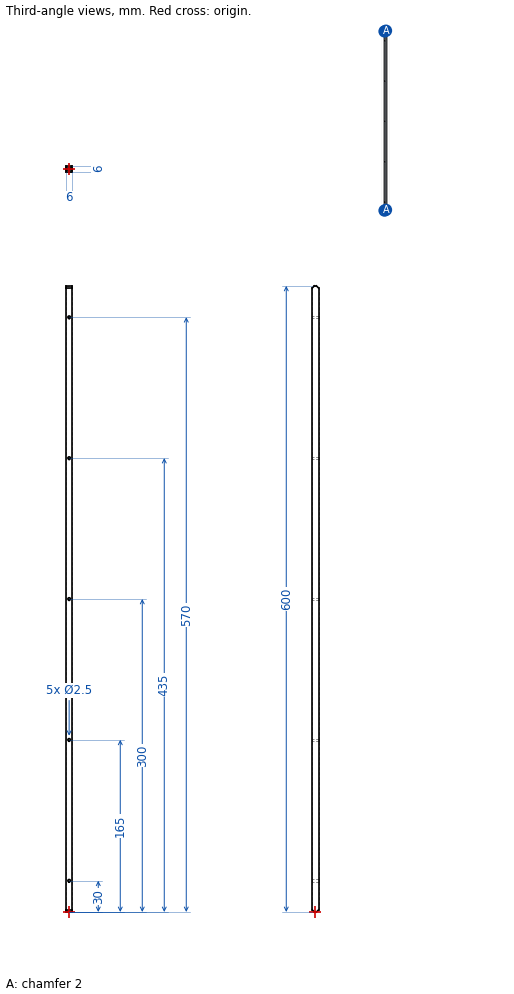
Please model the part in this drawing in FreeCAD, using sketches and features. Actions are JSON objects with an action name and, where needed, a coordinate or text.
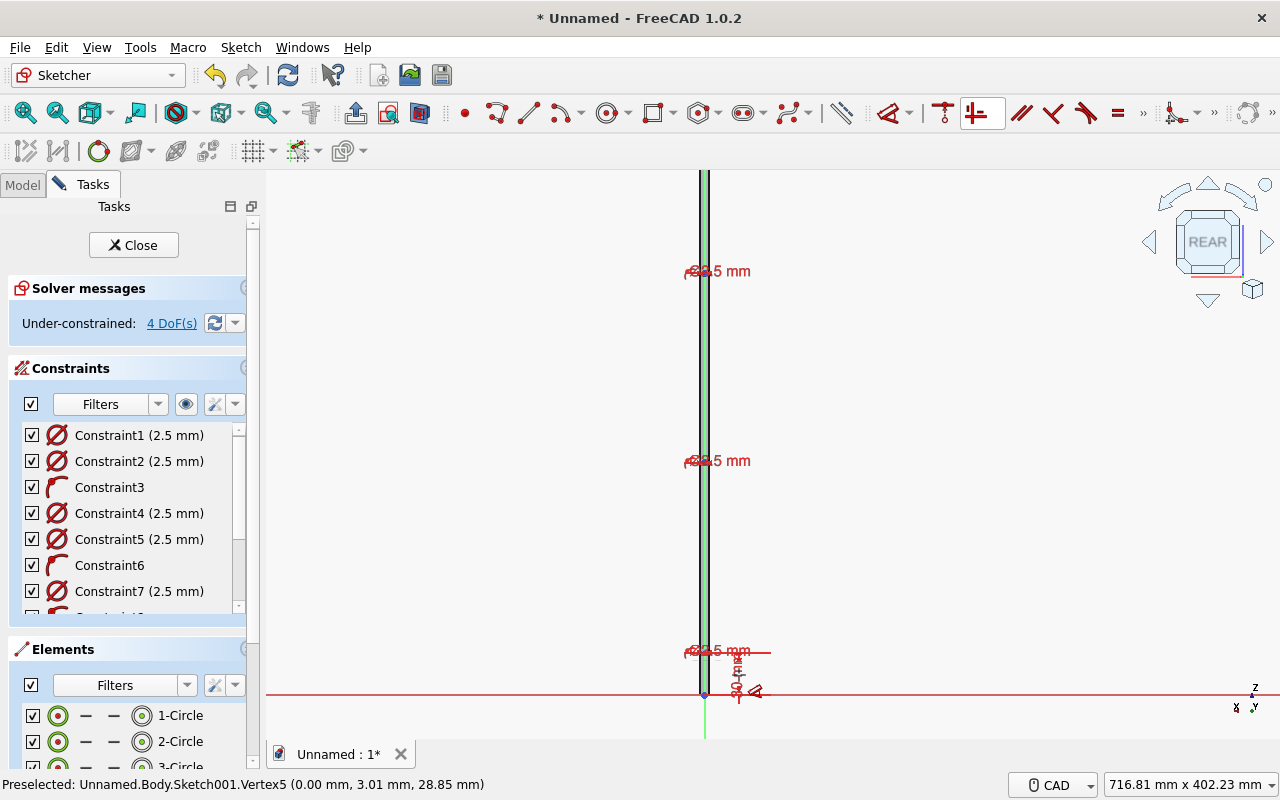
{"action": "left_click", "coordinate": [705, 463]}
{"action": "left_click", "coordinate": [739, 579]}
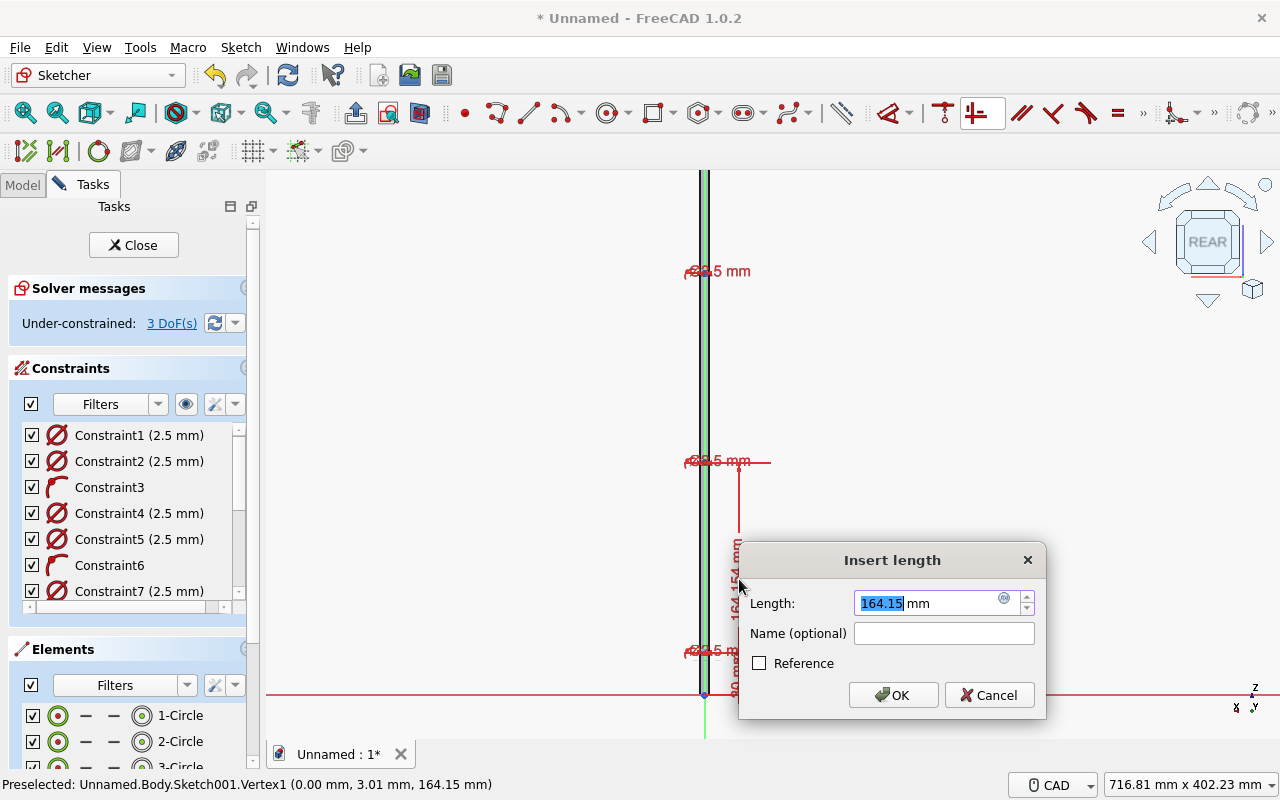
{"action": "type", "text": "165"}
{"action": "key", "text": "Return"}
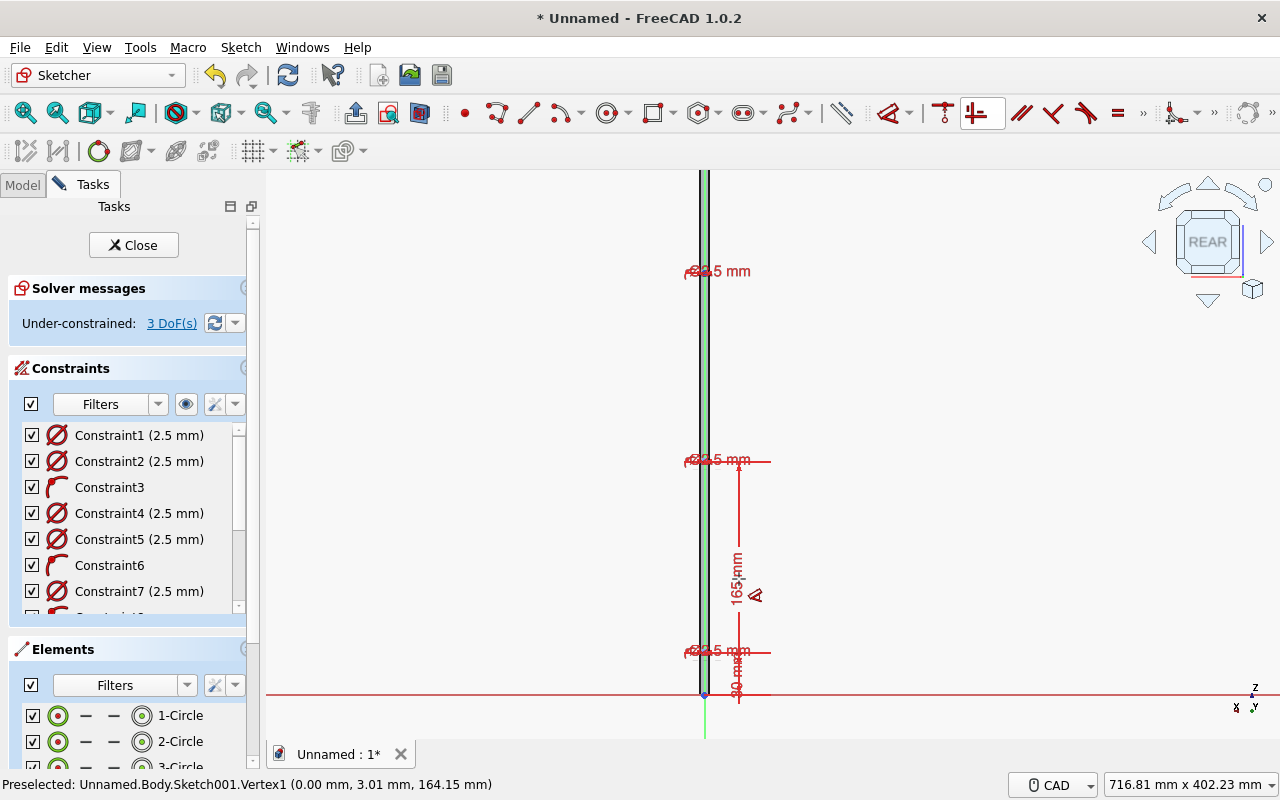
{"action": "left_click", "coordinate": [705, 273]}
{"action": "left_click", "coordinate": [739, 484]}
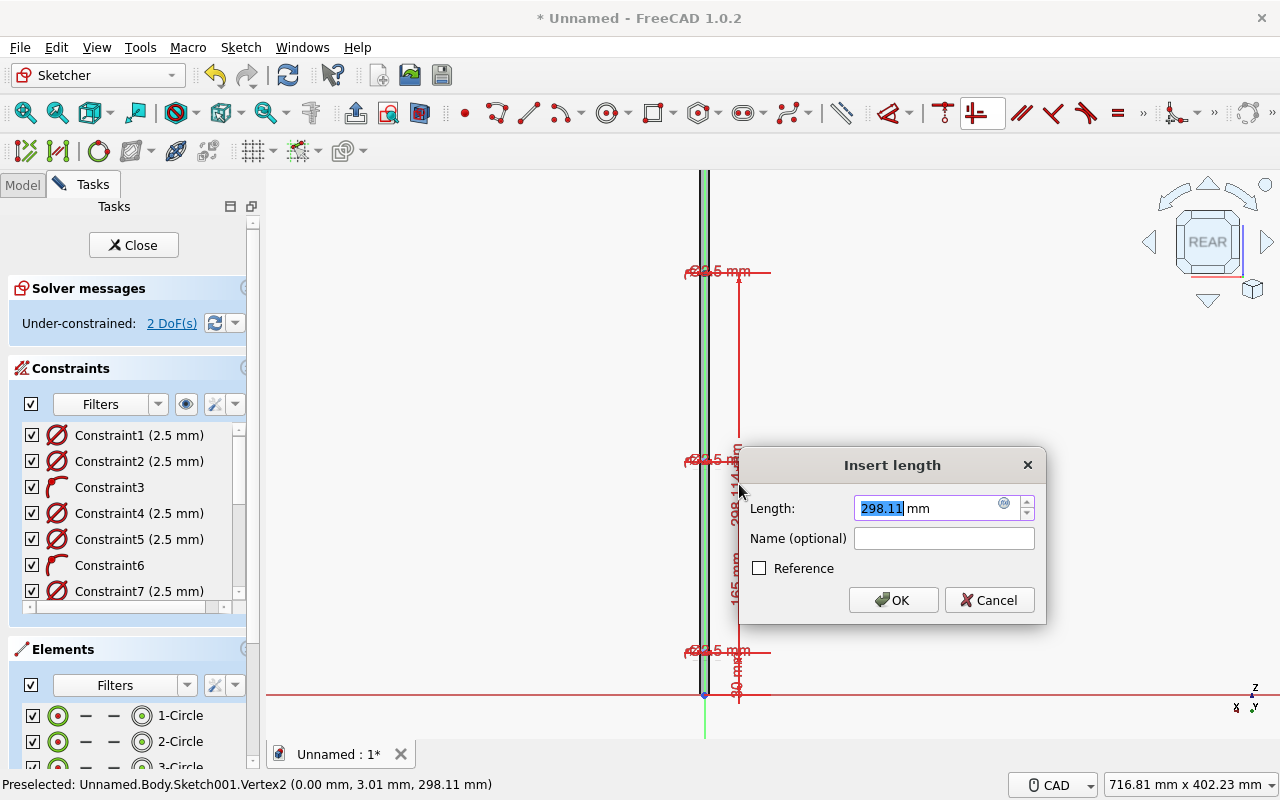
{"action": "type", "text": "300"}
{"action": "key", "text": "Return"}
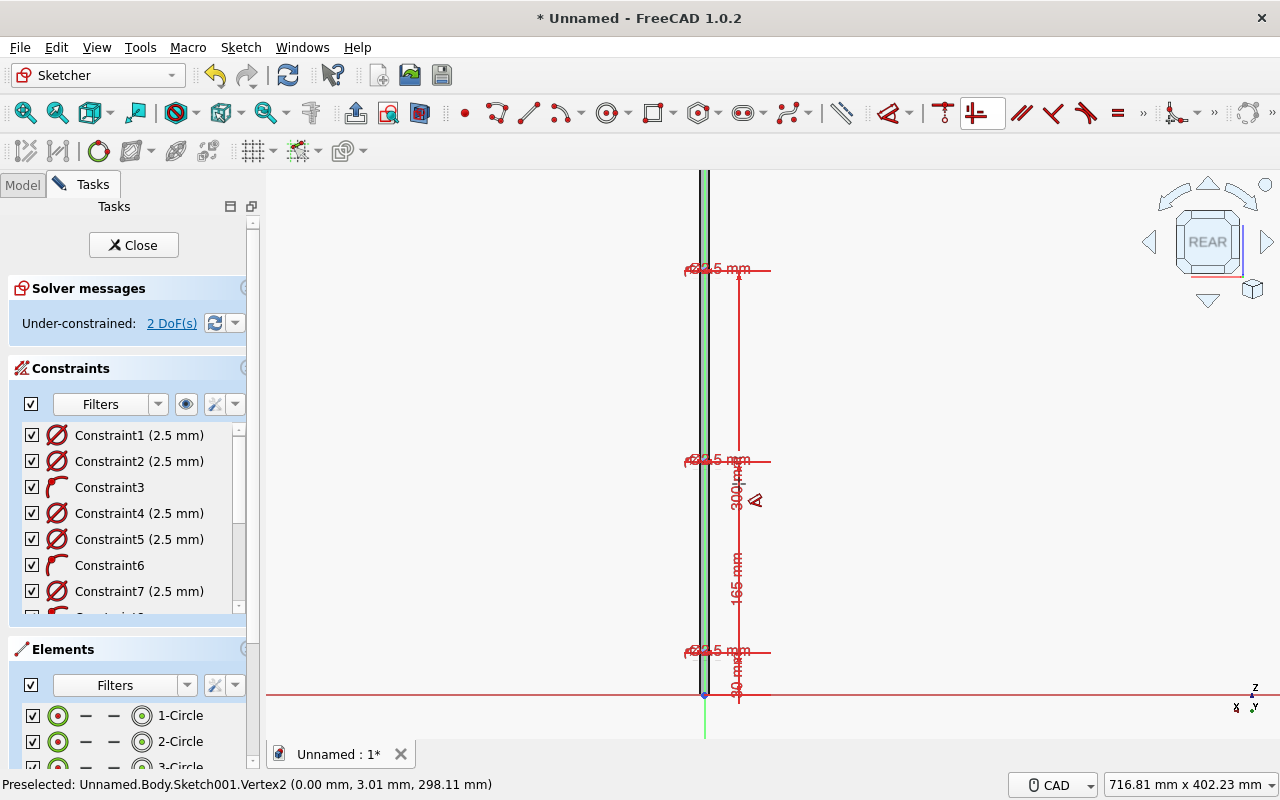
{"action": "scroll", "coordinate": [704, 588], "scroll_direction": "down", "scroll_amount": 4}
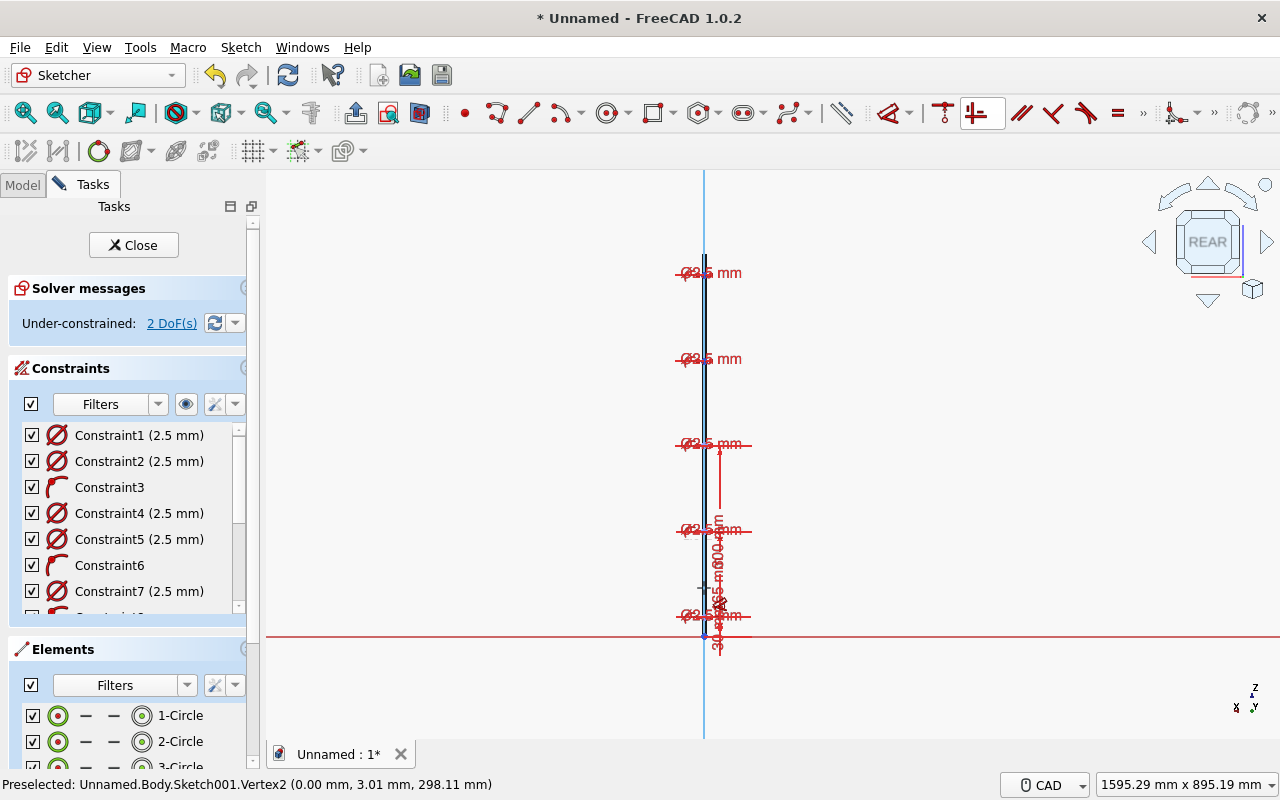
{"action": "left_click", "coordinate": [704, 361]}
{"action": "left_click", "coordinate": [738, 499]}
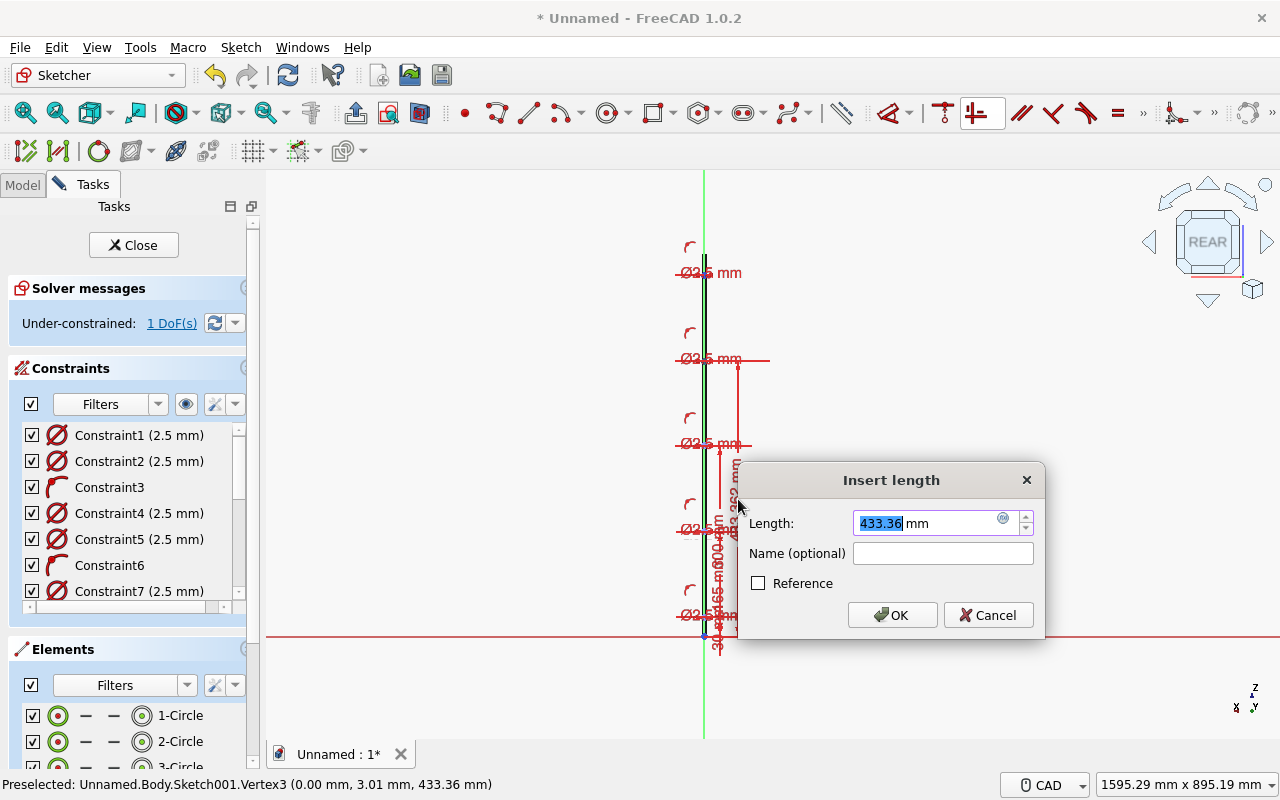
{"action": "type", "text": "435"}
{"action": "key", "text": "Return"}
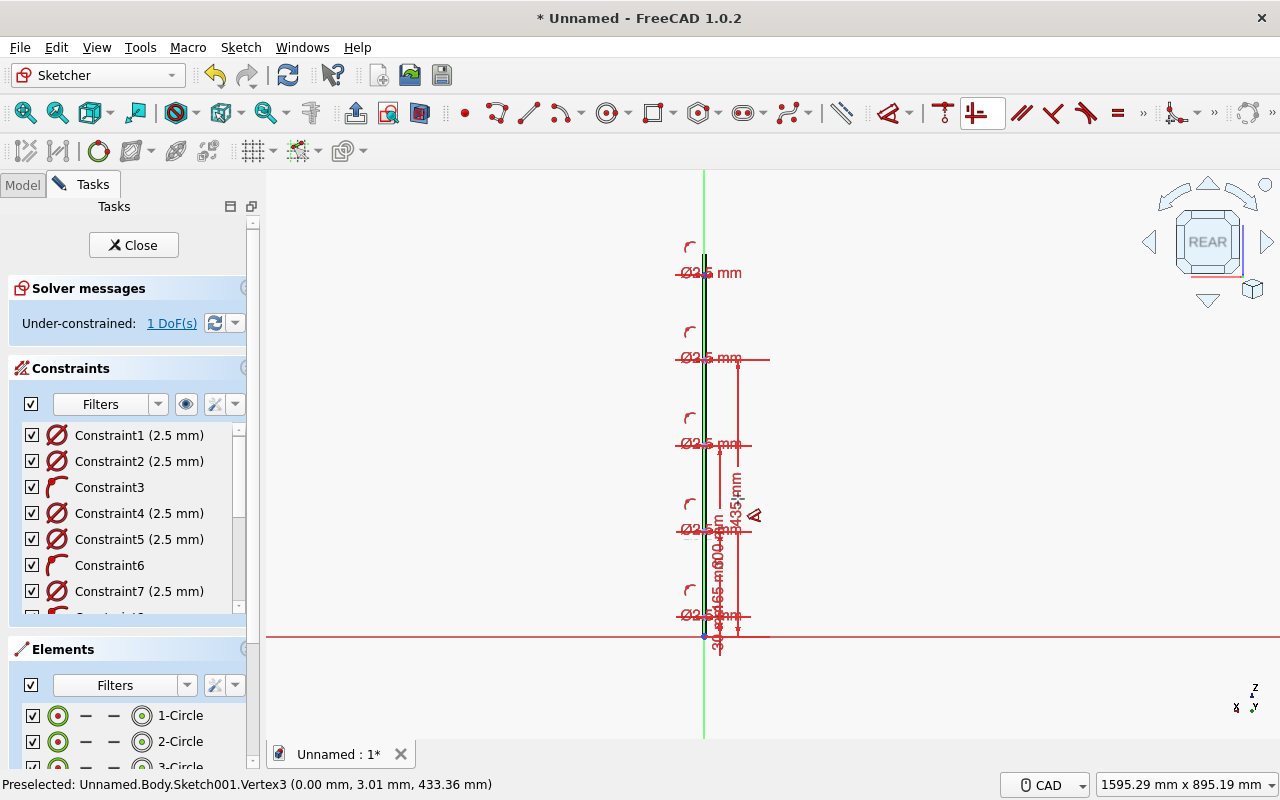
{"action": "left_click", "coordinate": [704, 275]}
{"action": "left_click", "coordinate": [738, 456]}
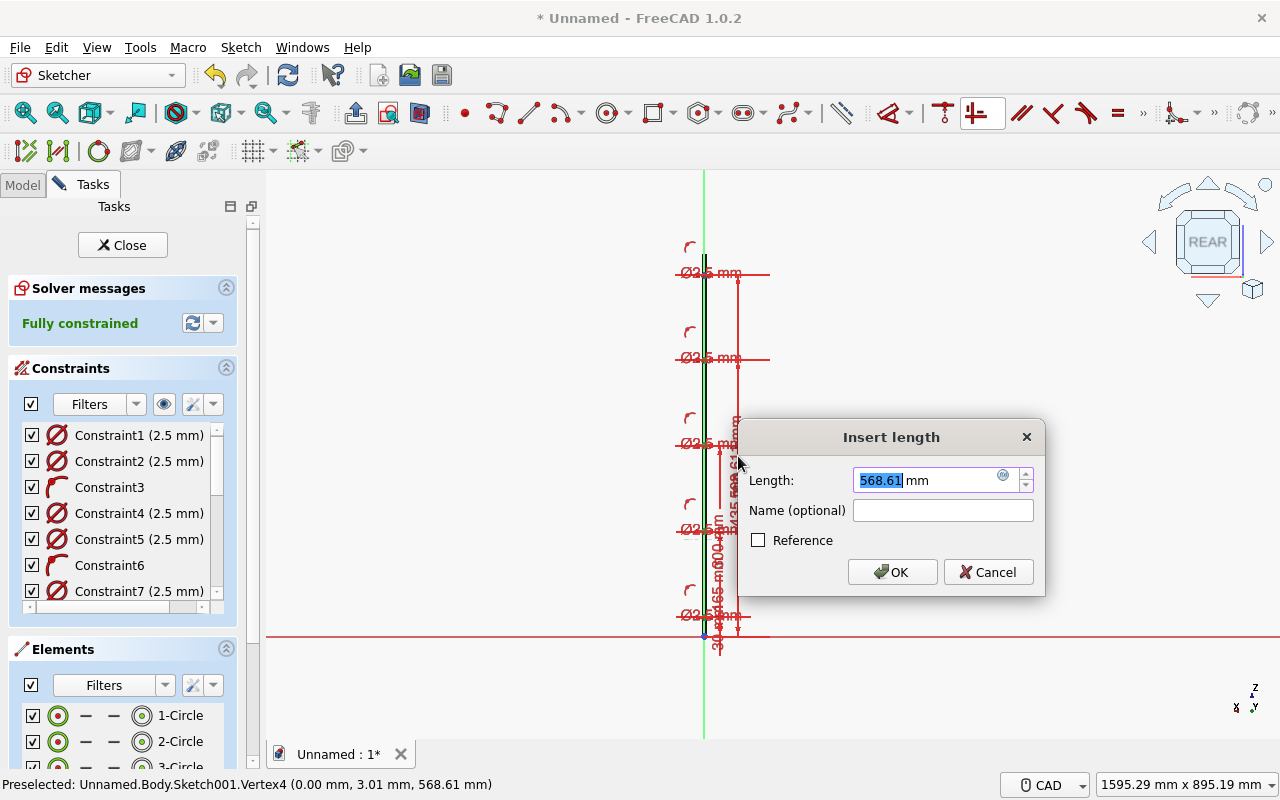
{"action": "type", "text": "570"}
{"action": "key", "text": "Return"}
{"action": "key", "text": "Escape"}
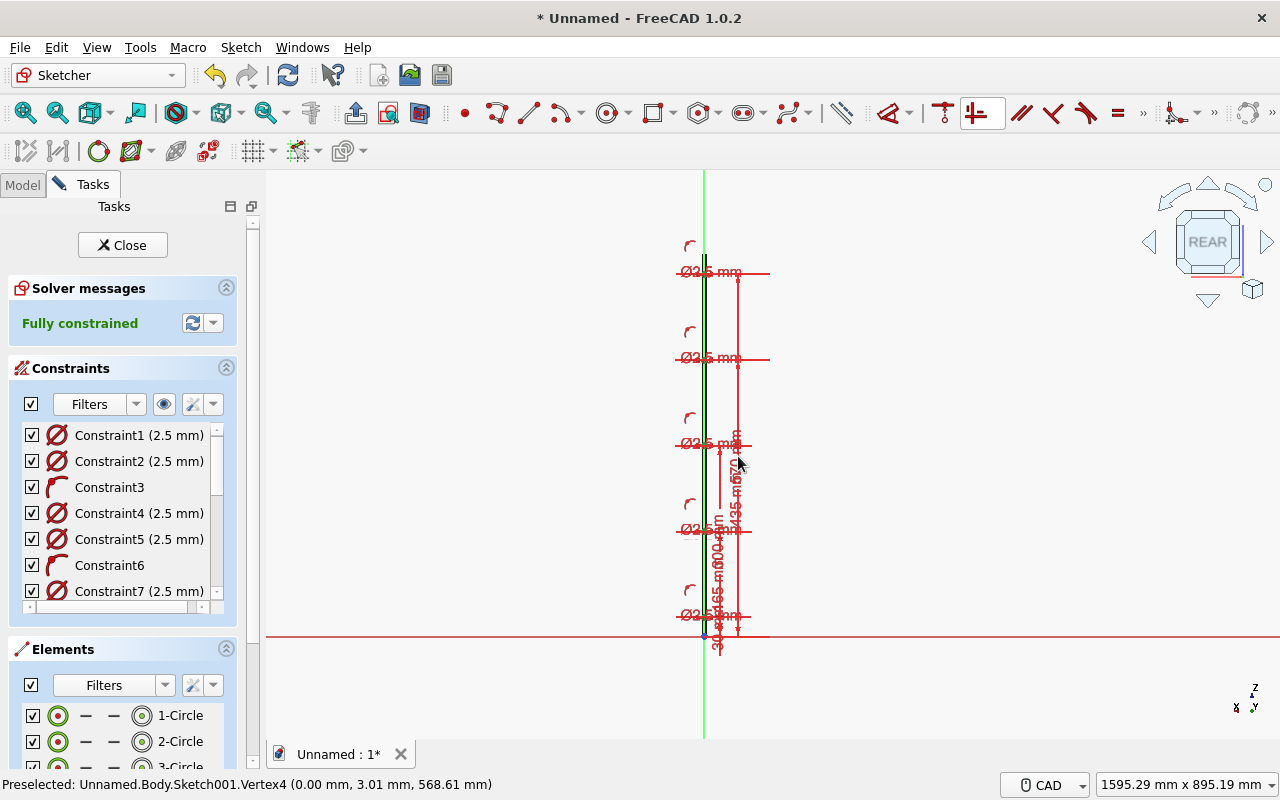
{"action": "left_click", "coordinate": [123, 245]}